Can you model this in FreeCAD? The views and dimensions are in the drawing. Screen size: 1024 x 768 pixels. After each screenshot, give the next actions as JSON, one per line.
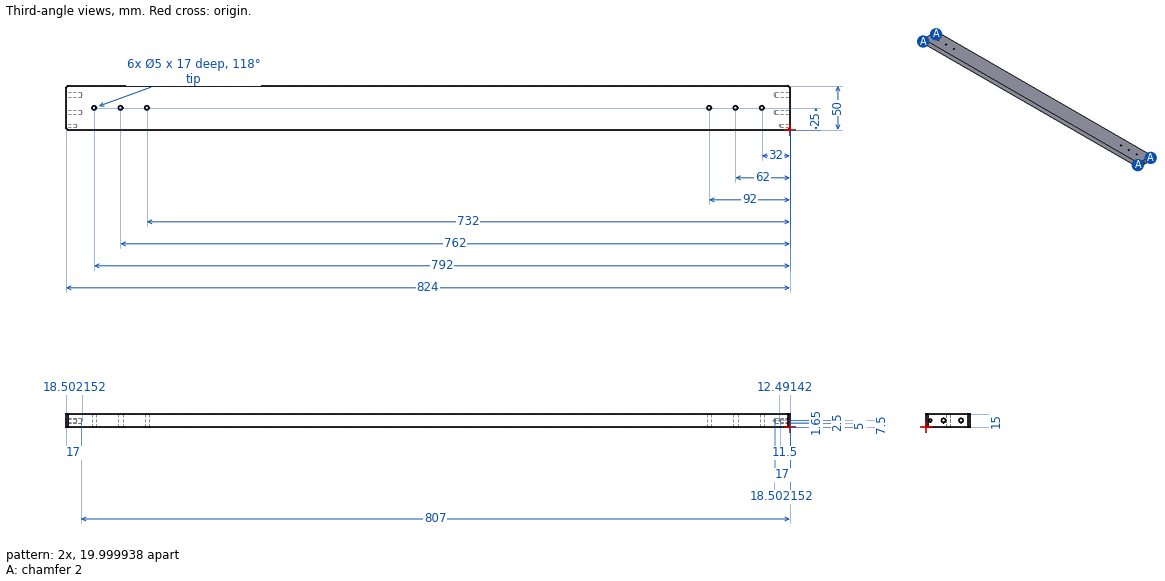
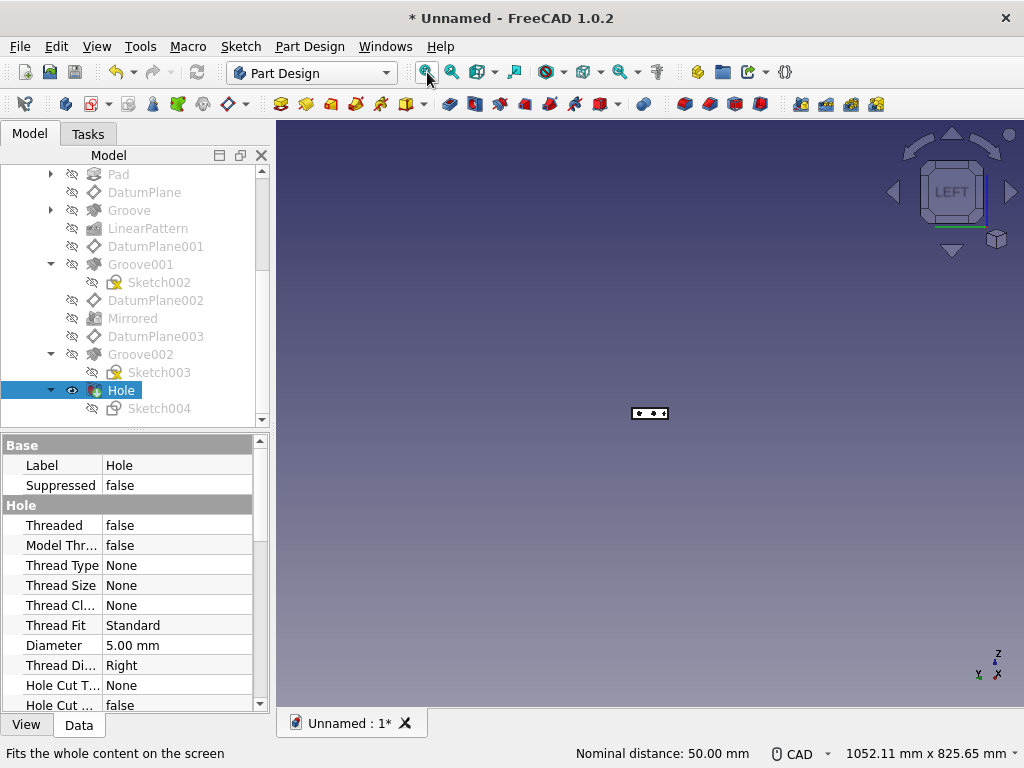
{"action": "scroll", "coordinate": [668, 412], "scroll_direction": "up", "scroll_amount": 7}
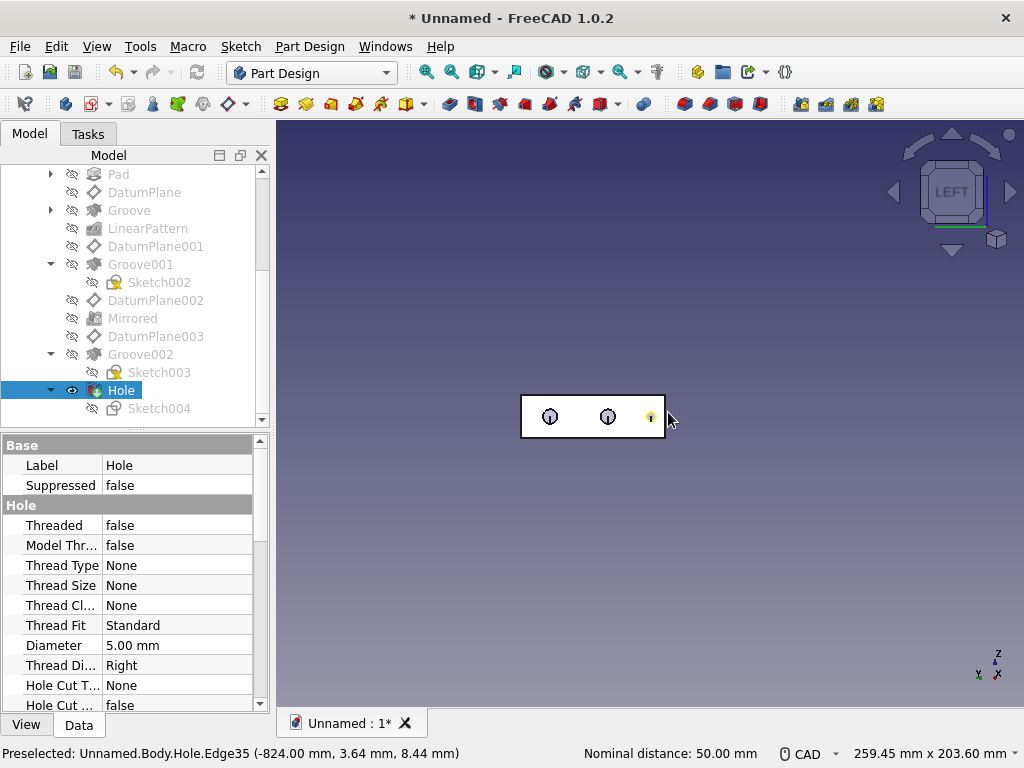
{"action": "left_click", "coordinate": [665, 416], "text": "ctrl"}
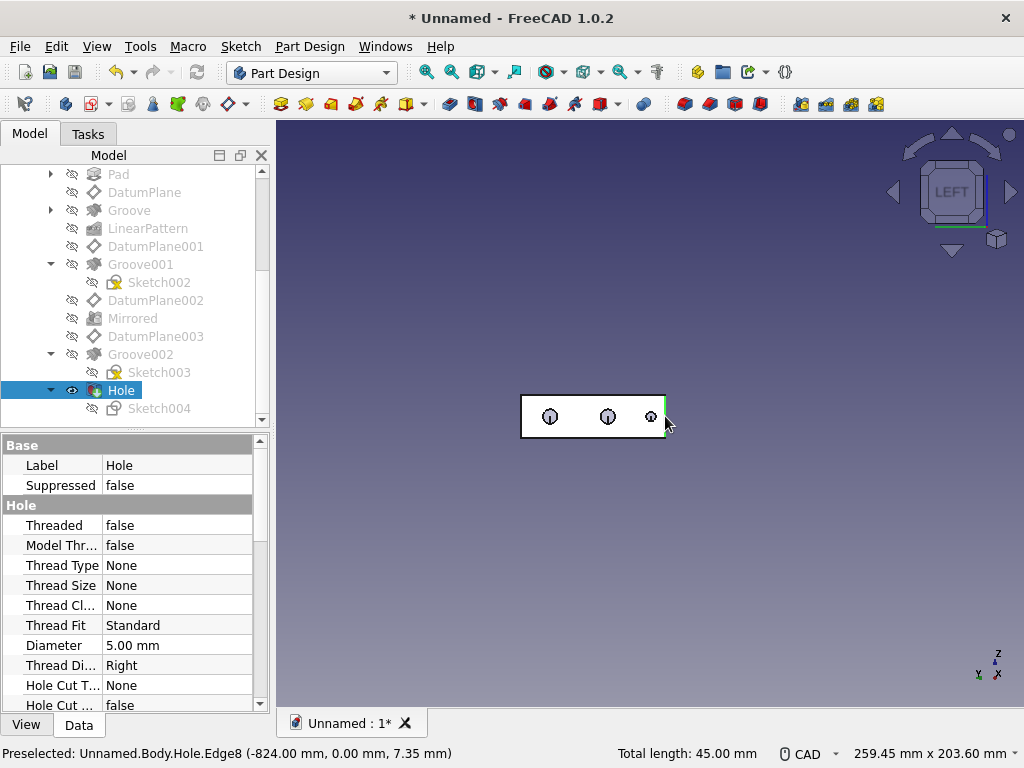
{"action": "left_click", "coordinate": [521, 416], "text": "ctrl"}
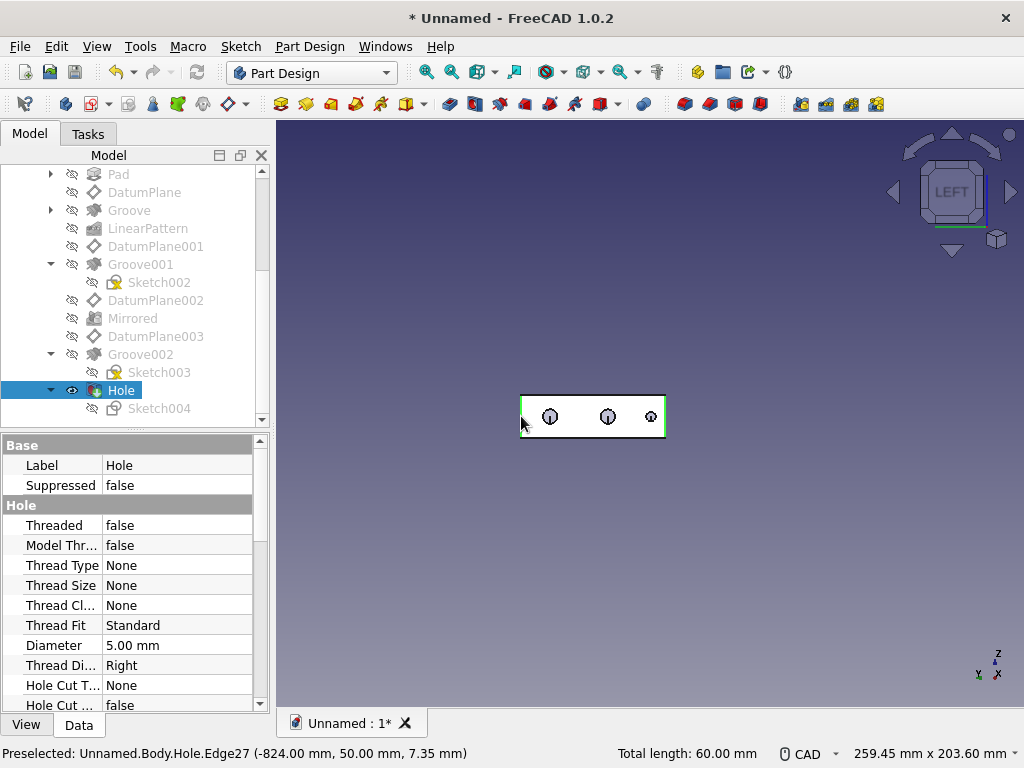
{"action": "left_click", "coordinate": [710, 104]}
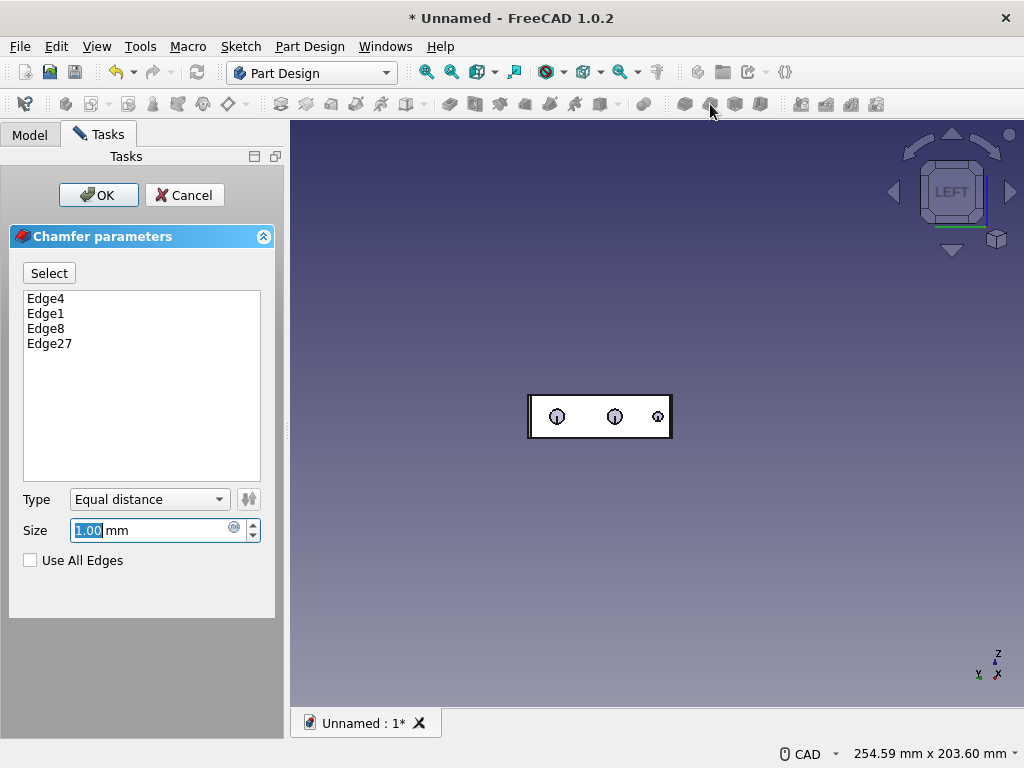
{"action": "type", "text": "2"}
{"action": "key", "text": "Tab"}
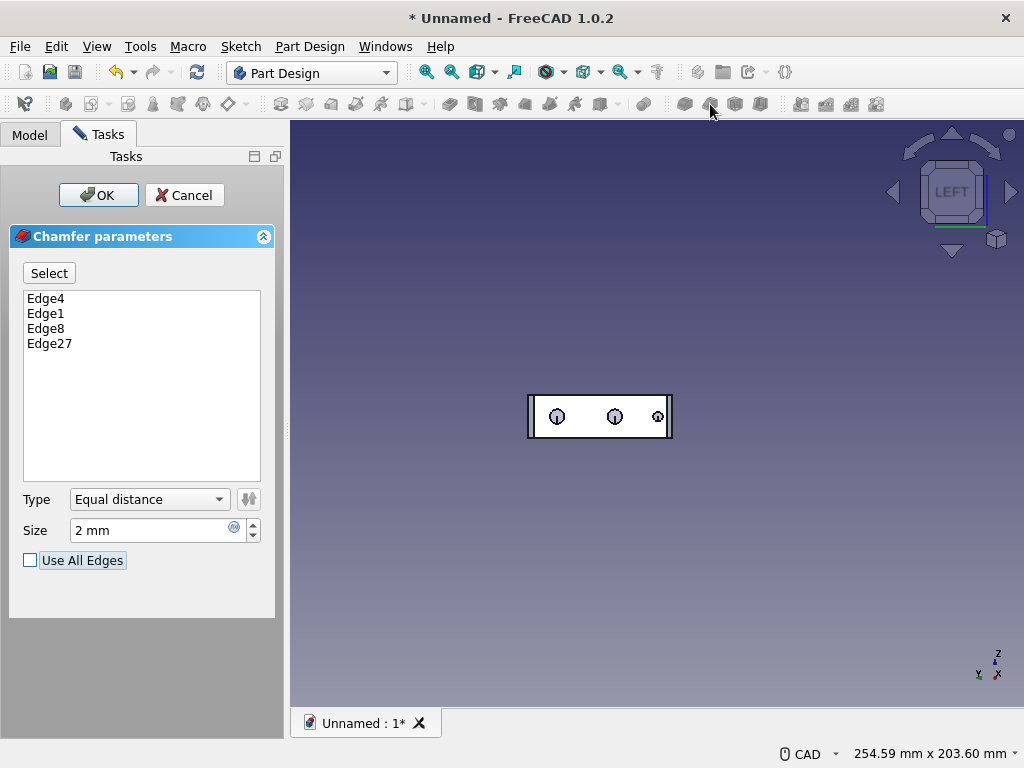
{"action": "left_click", "coordinate": [99, 195]}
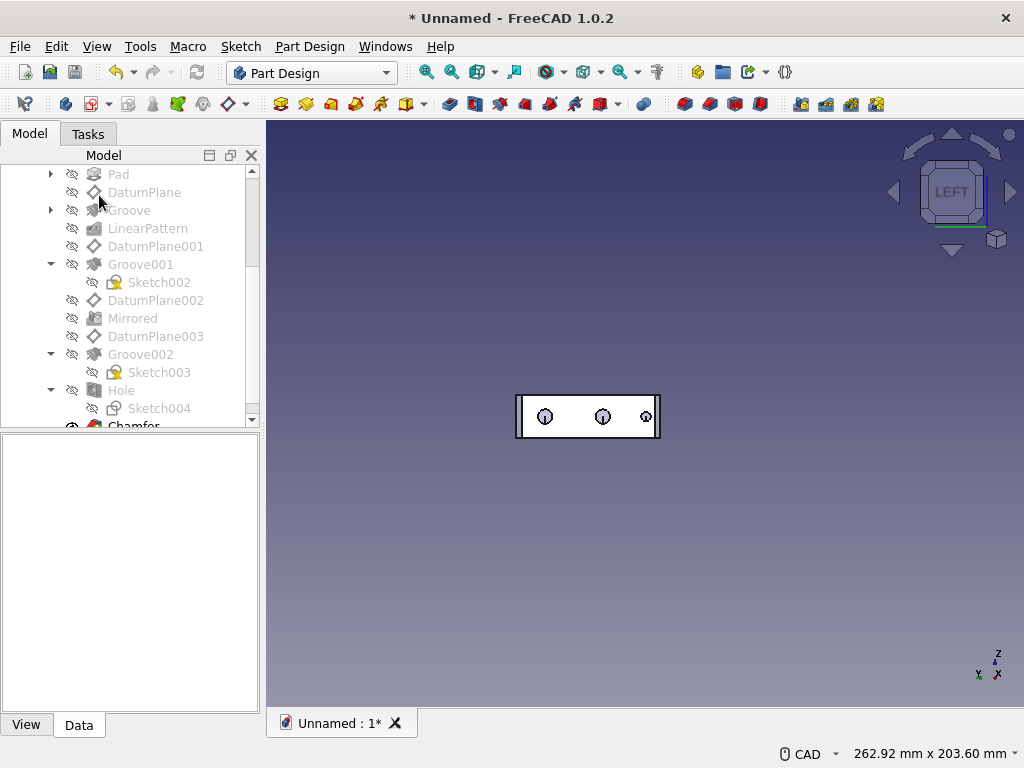
{"action": "key", "text": "0"}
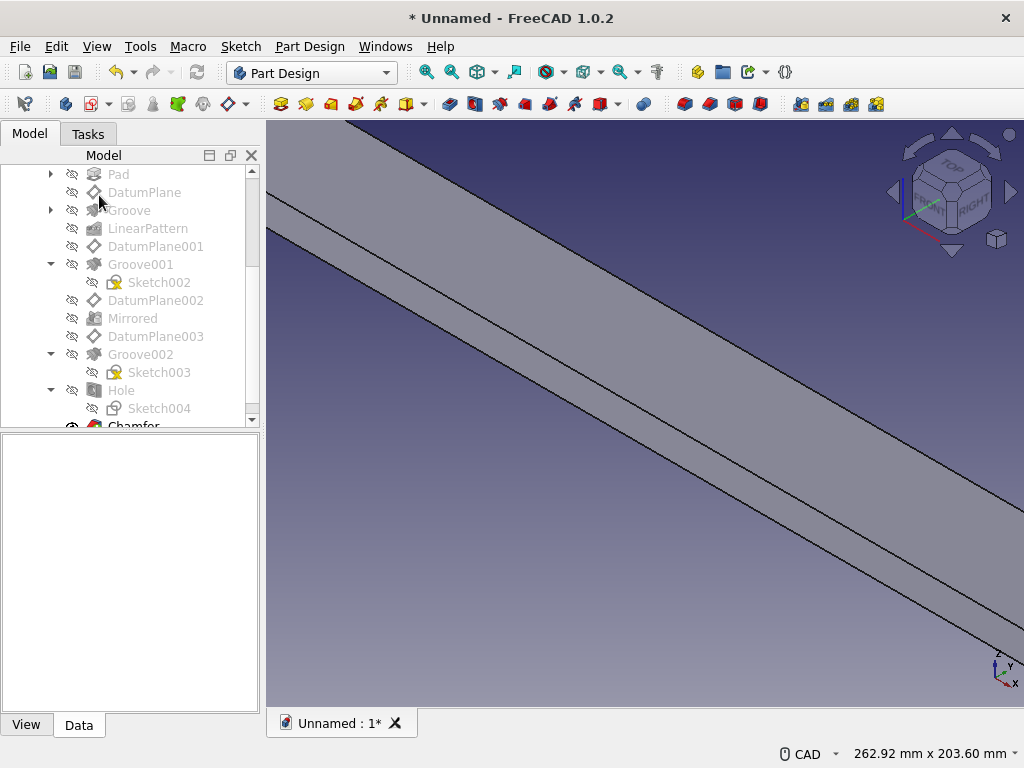
{"action": "left_click", "coordinate": [427, 72]}